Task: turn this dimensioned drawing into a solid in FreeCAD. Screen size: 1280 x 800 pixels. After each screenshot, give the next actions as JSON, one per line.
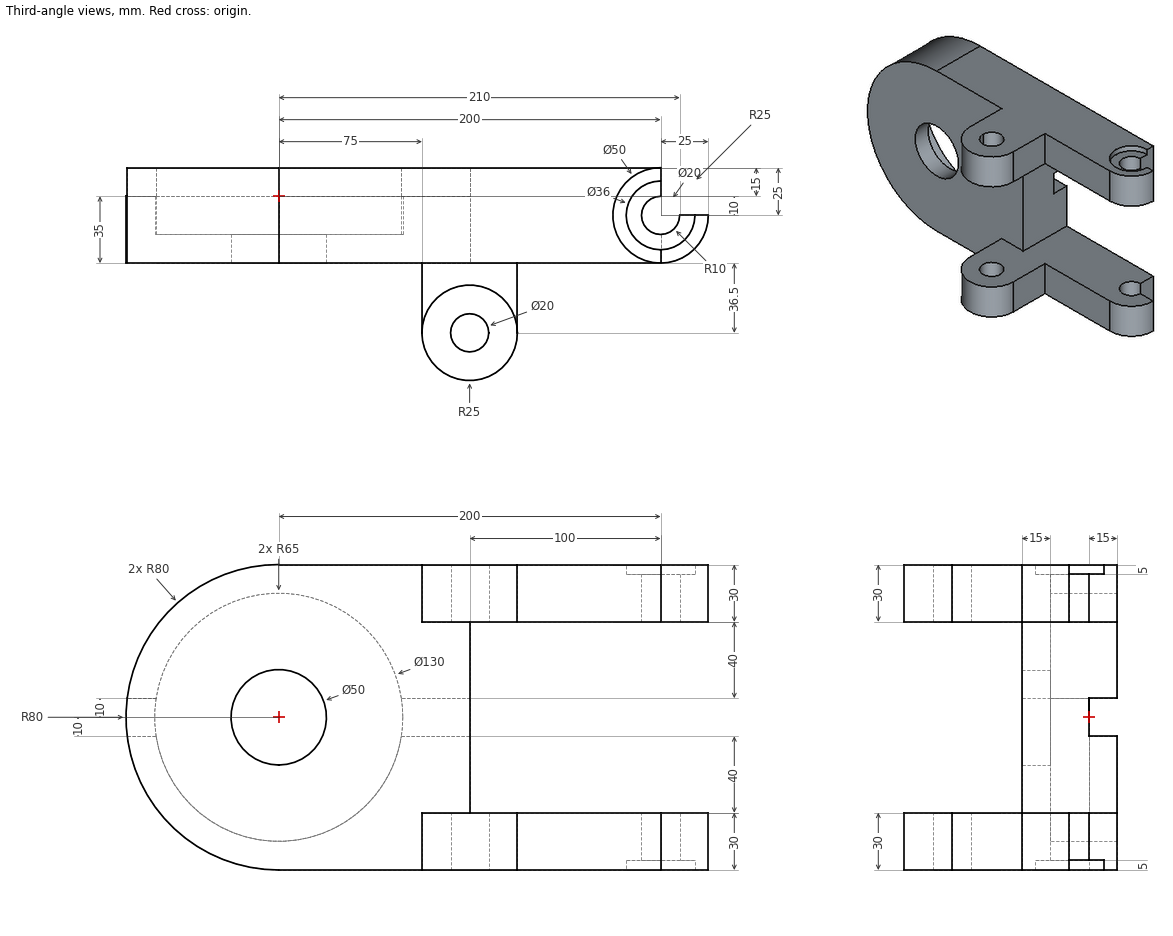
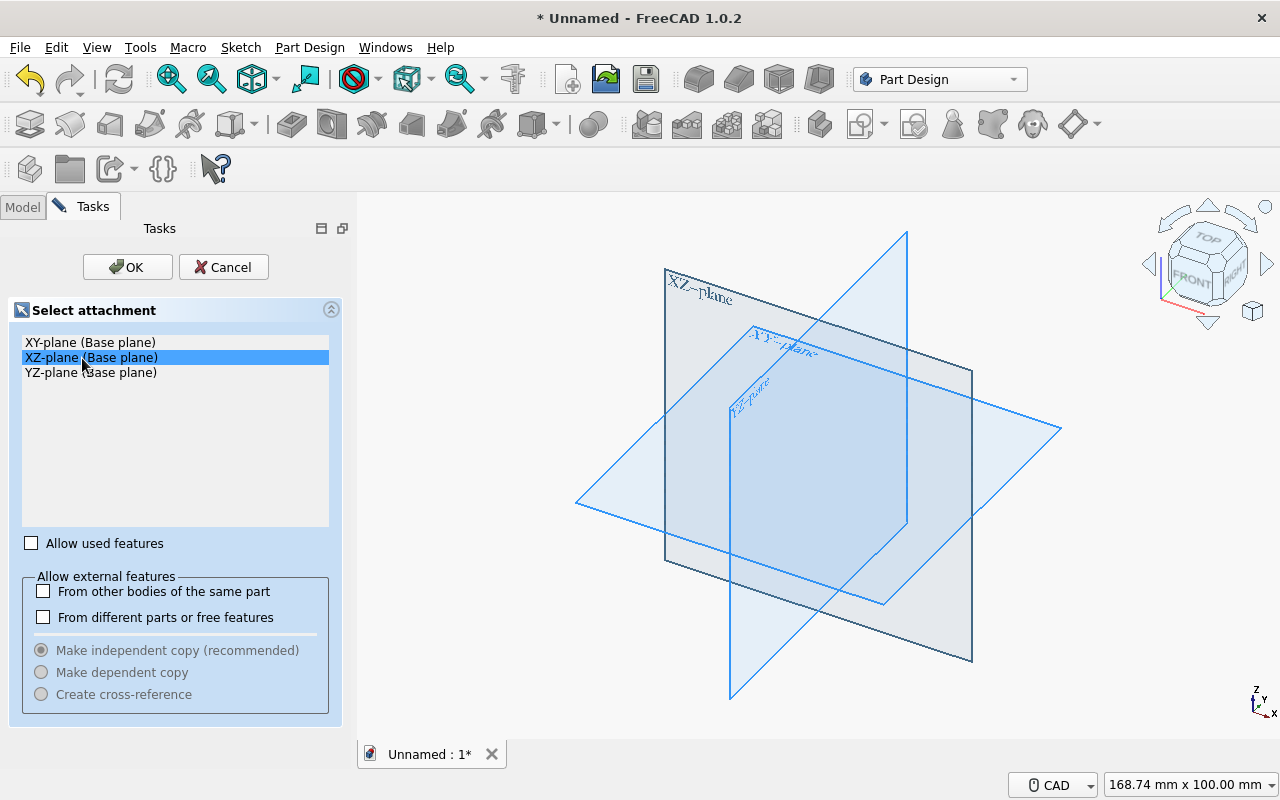
{"action": "left_click", "coordinate": [128, 267]}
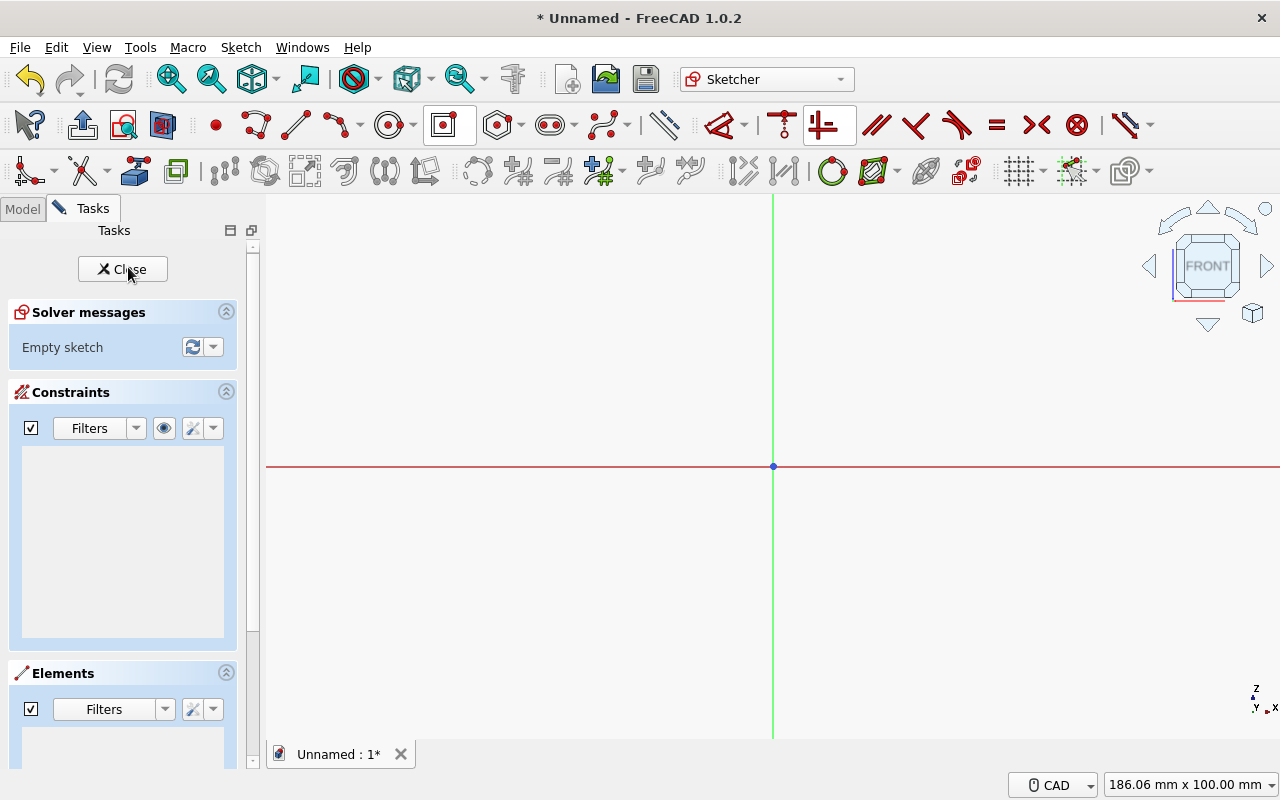
{"action": "scroll", "coordinate": [473, 466], "scroll_direction": "down", "scroll_amount": 5}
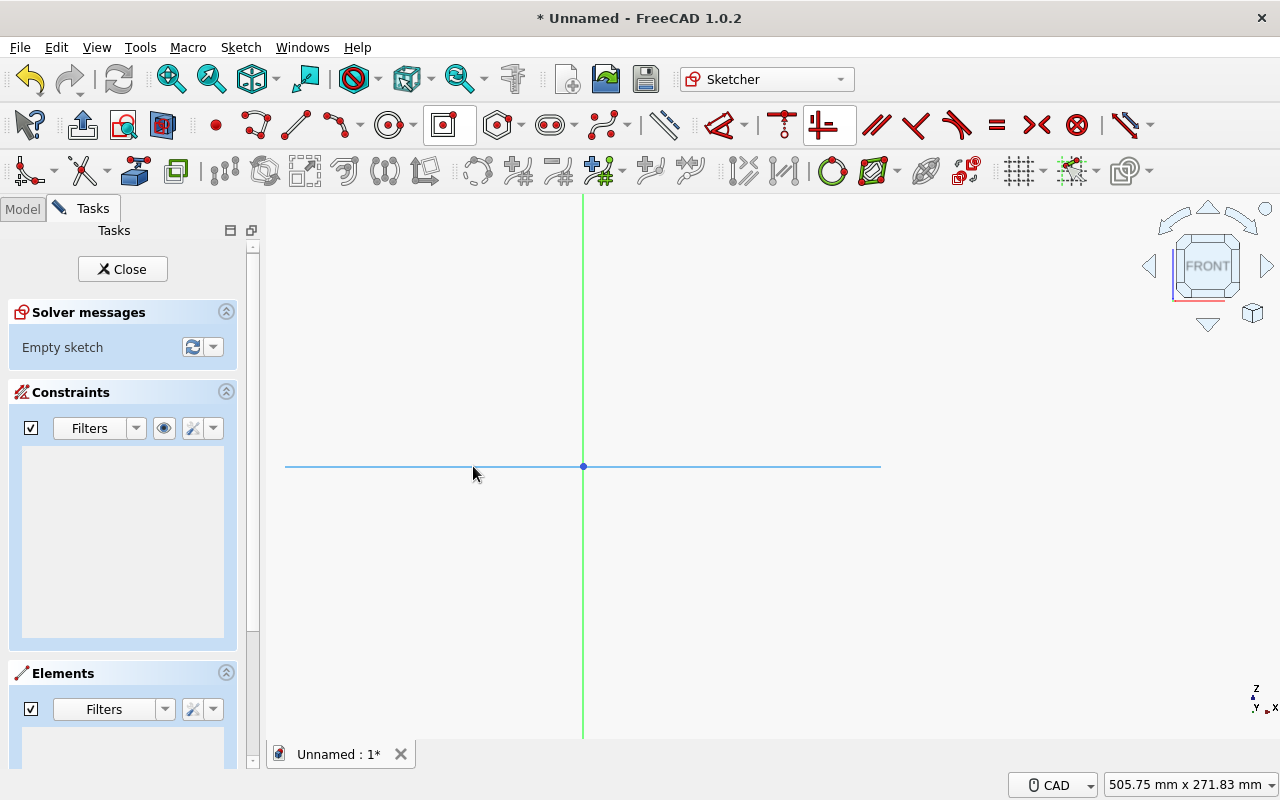
{"action": "left_click", "coordinate": [296, 126]}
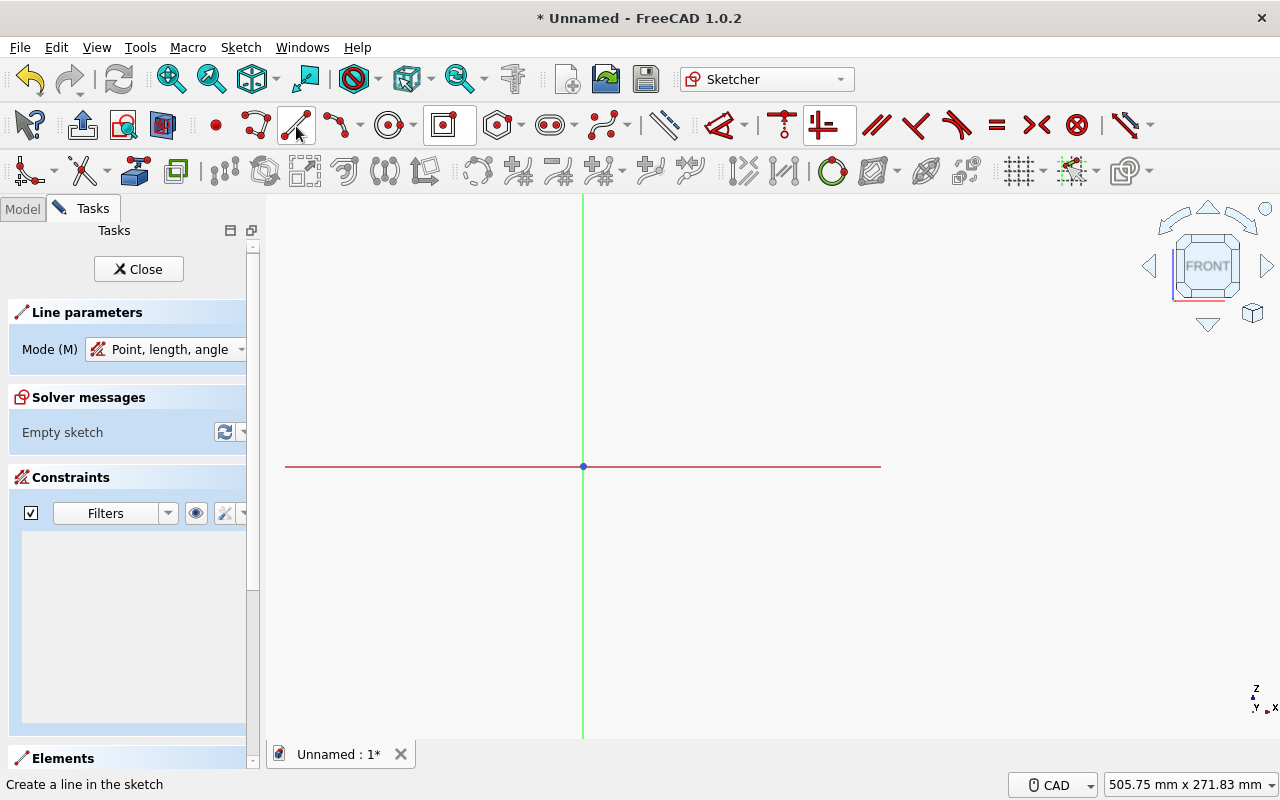
{"action": "left_click", "coordinate": [455, 446]}
{"action": "left_click", "coordinate": [424, 446]}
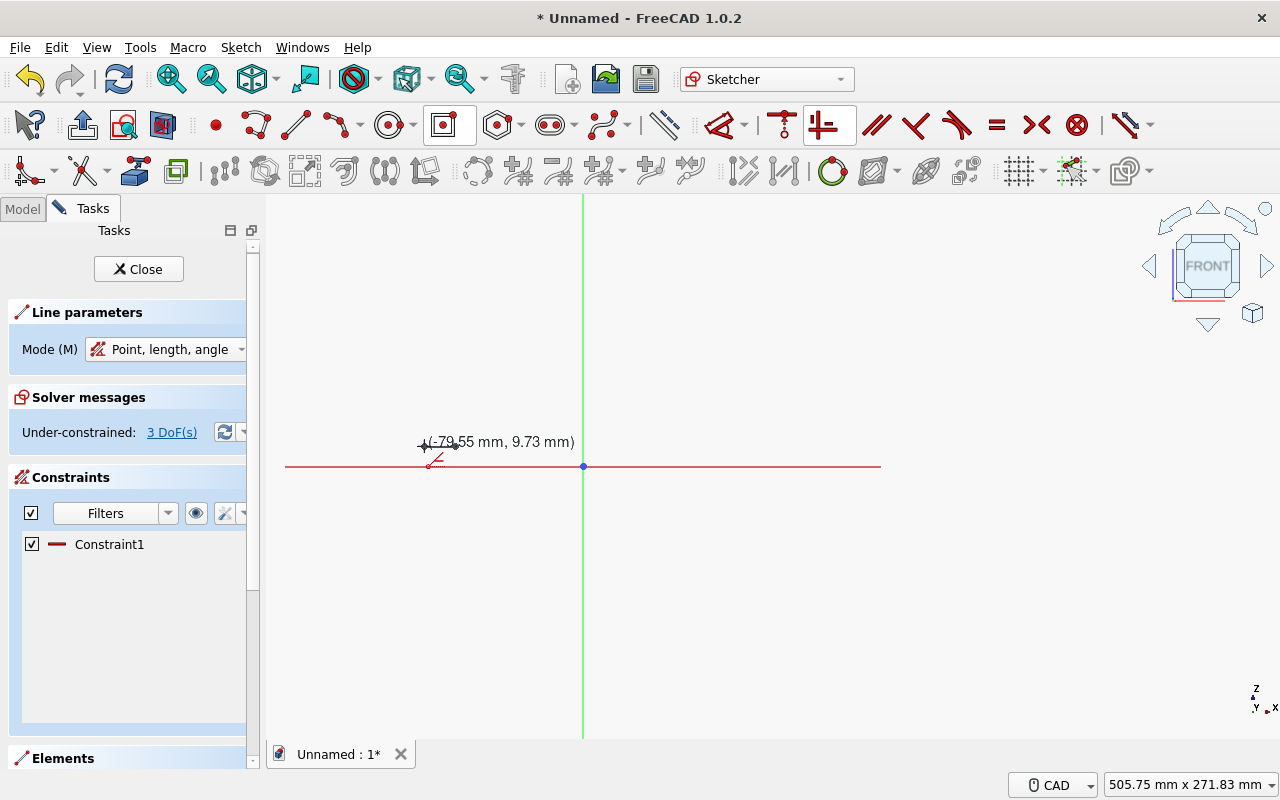
{"action": "key", "text": "g m"}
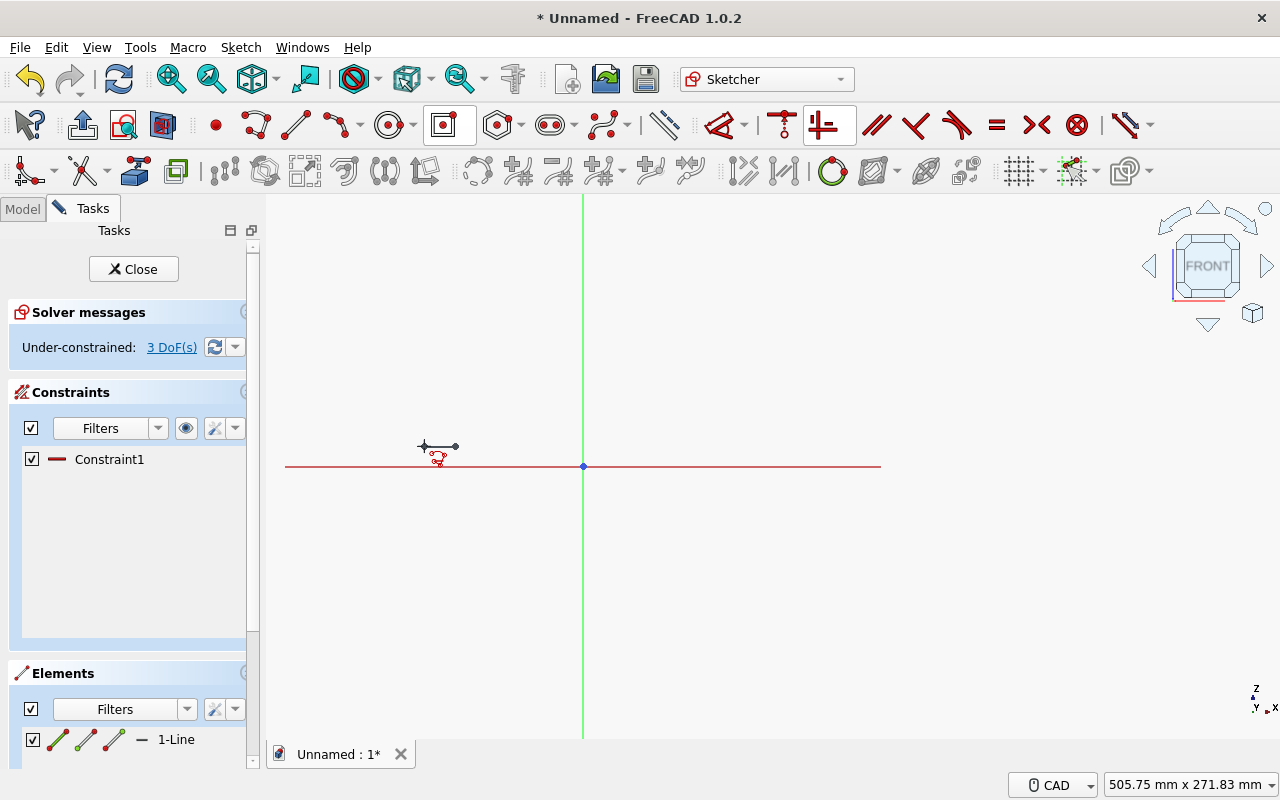
{"action": "left_click", "coordinate": [583, 306]}
{"action": "left_click", "coordinate": [984, 306]}
{"action": "left_click", "coordinate": [984, 366]}
{"action": "left_click", "coordinate": [784, 366]}
{"action": "left_click", "coordinate": [784, 446]}
{"action": "left_click", "coordinate": [712, 446]}
{"action": "right_click", "coordinate": [712, 446]}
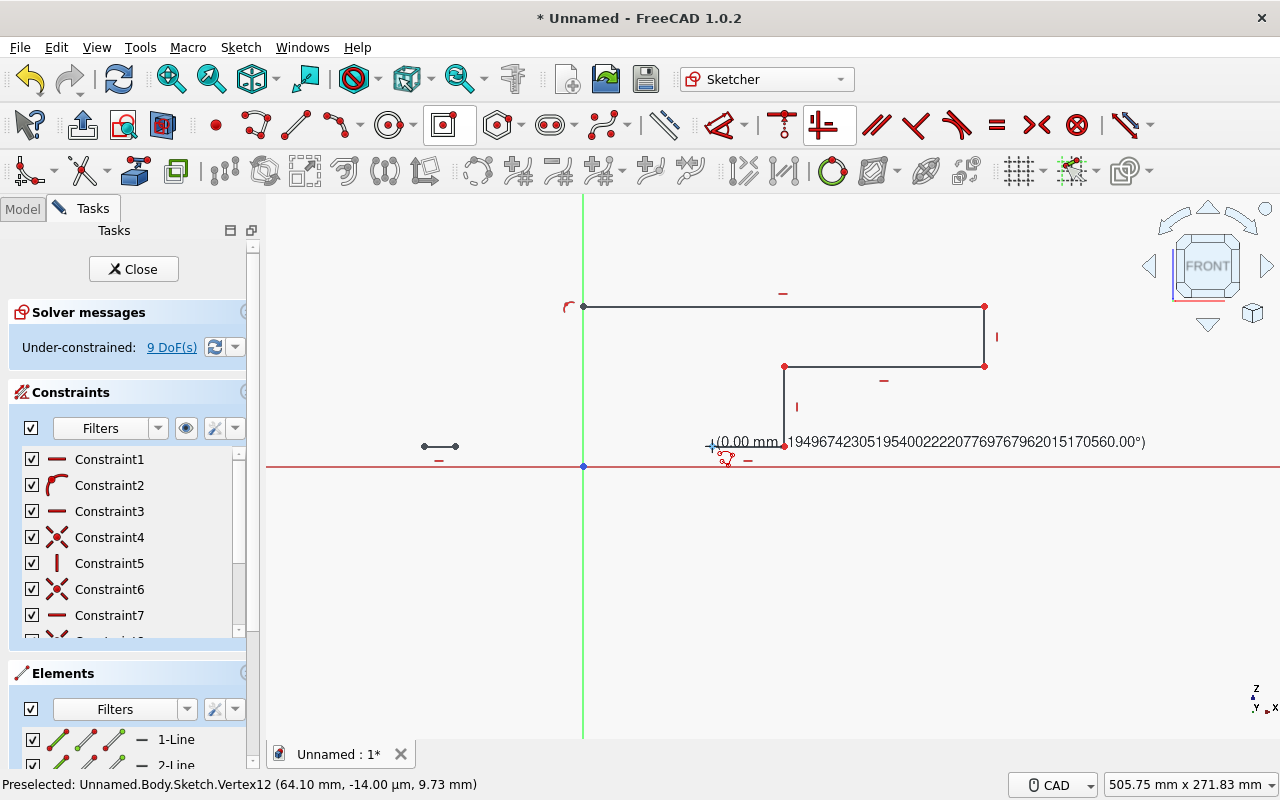
{"action": "left_click", "coordinate": [336, 126]}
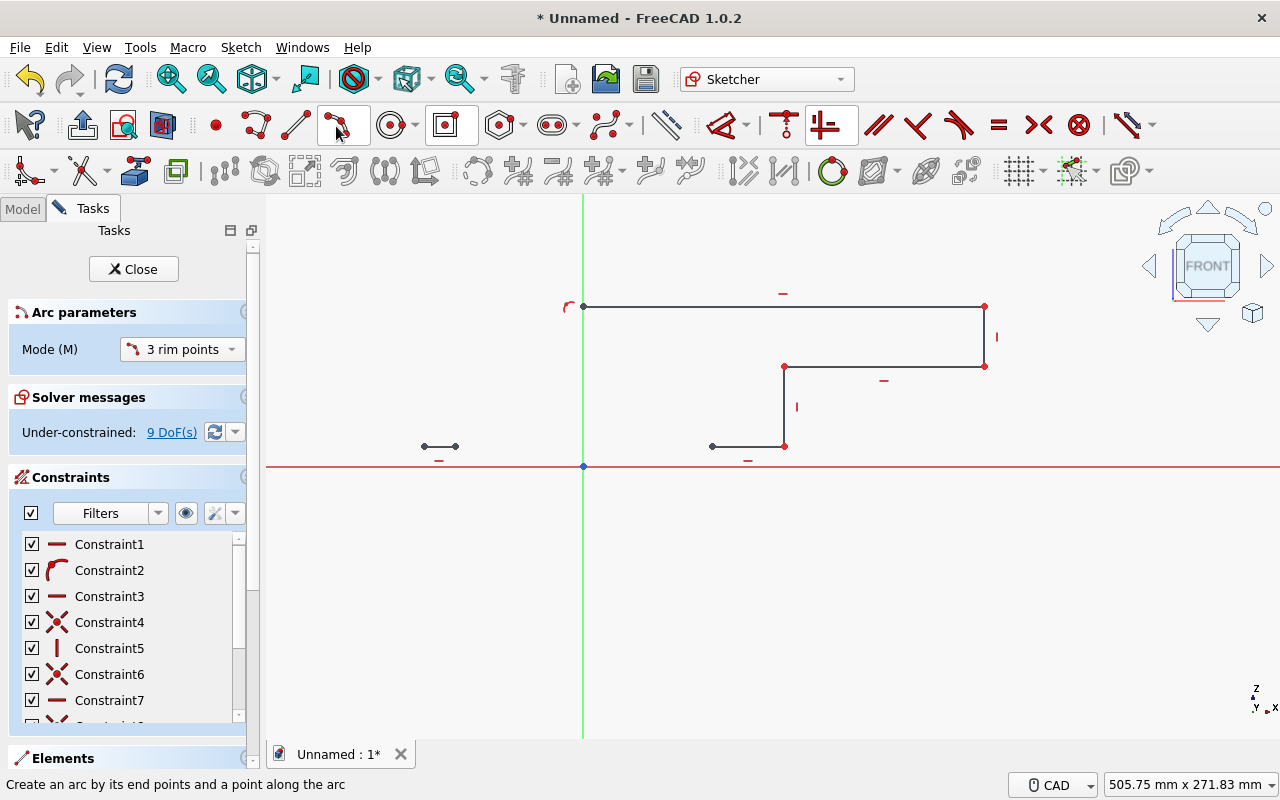
{"action": "left_click", "coordinate": [424, 447]}
{"action": "left_click", "coordinate": [583, 307]}
{"action": "left_click", "coordinate": [477, 346]}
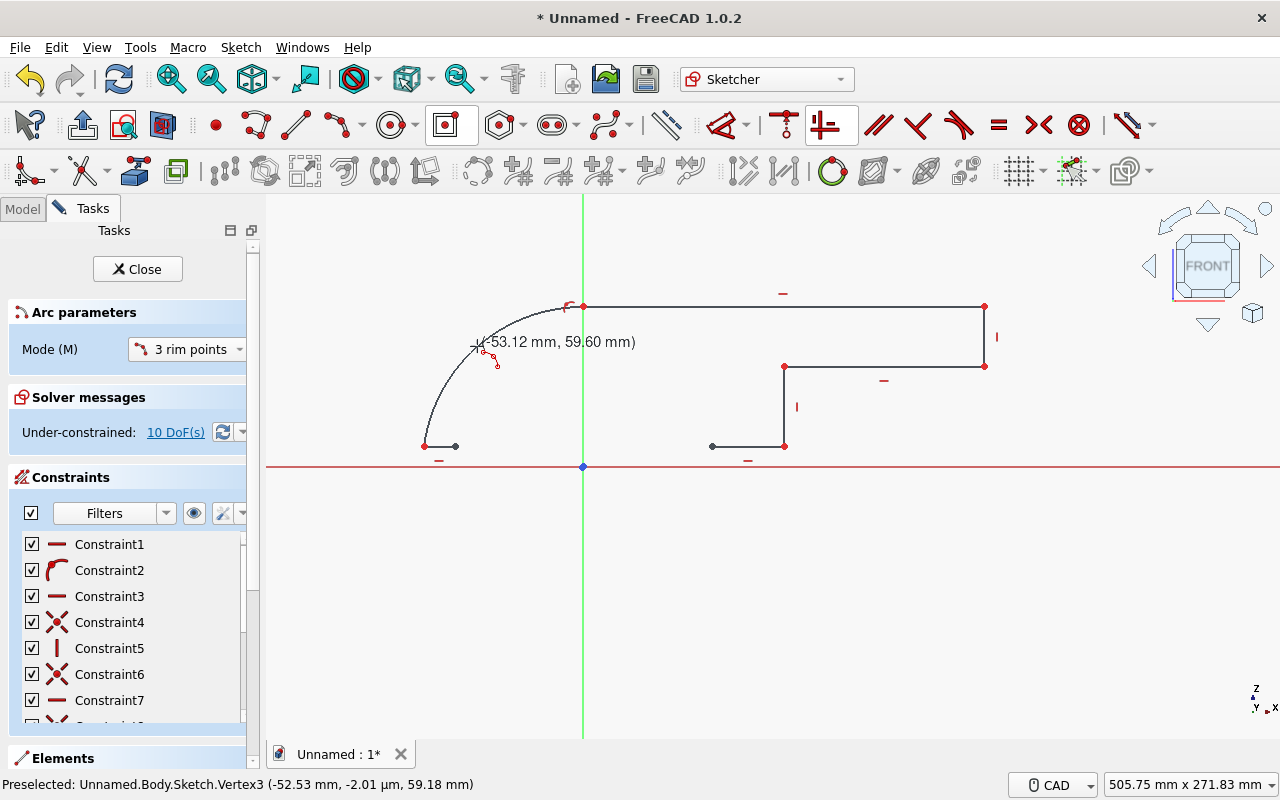
{"action": "left_click", "coordinate": [712, 447]}
{"action": "left_click", "coordinate": [455, 447]}
{"action": "left_click", "coordinate": [620, 341]}